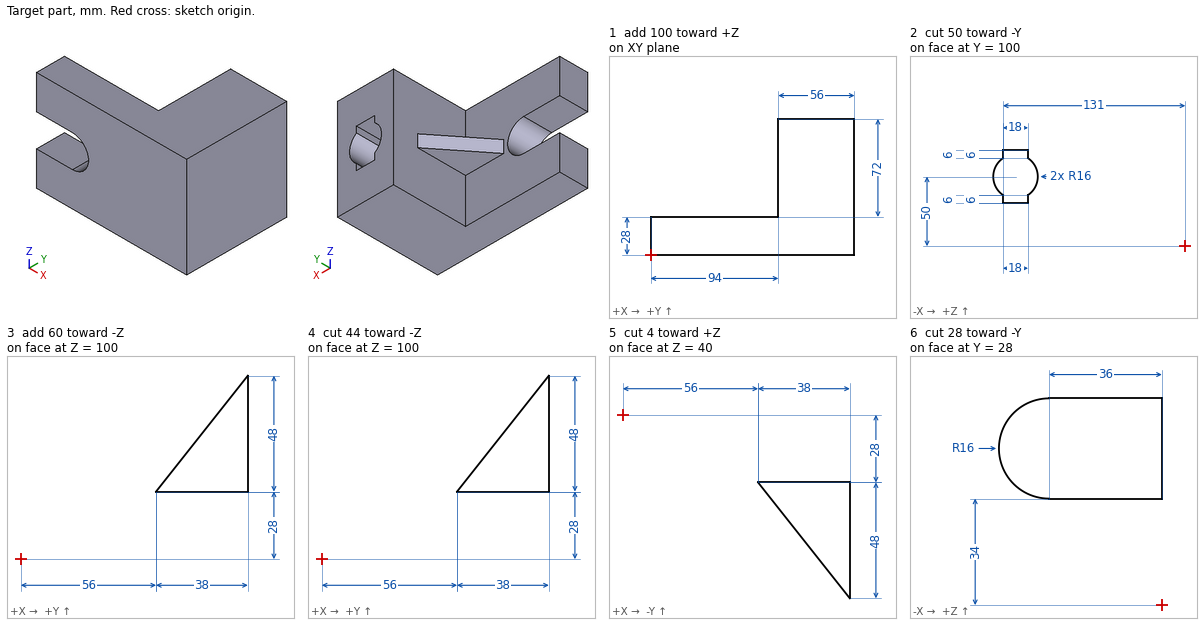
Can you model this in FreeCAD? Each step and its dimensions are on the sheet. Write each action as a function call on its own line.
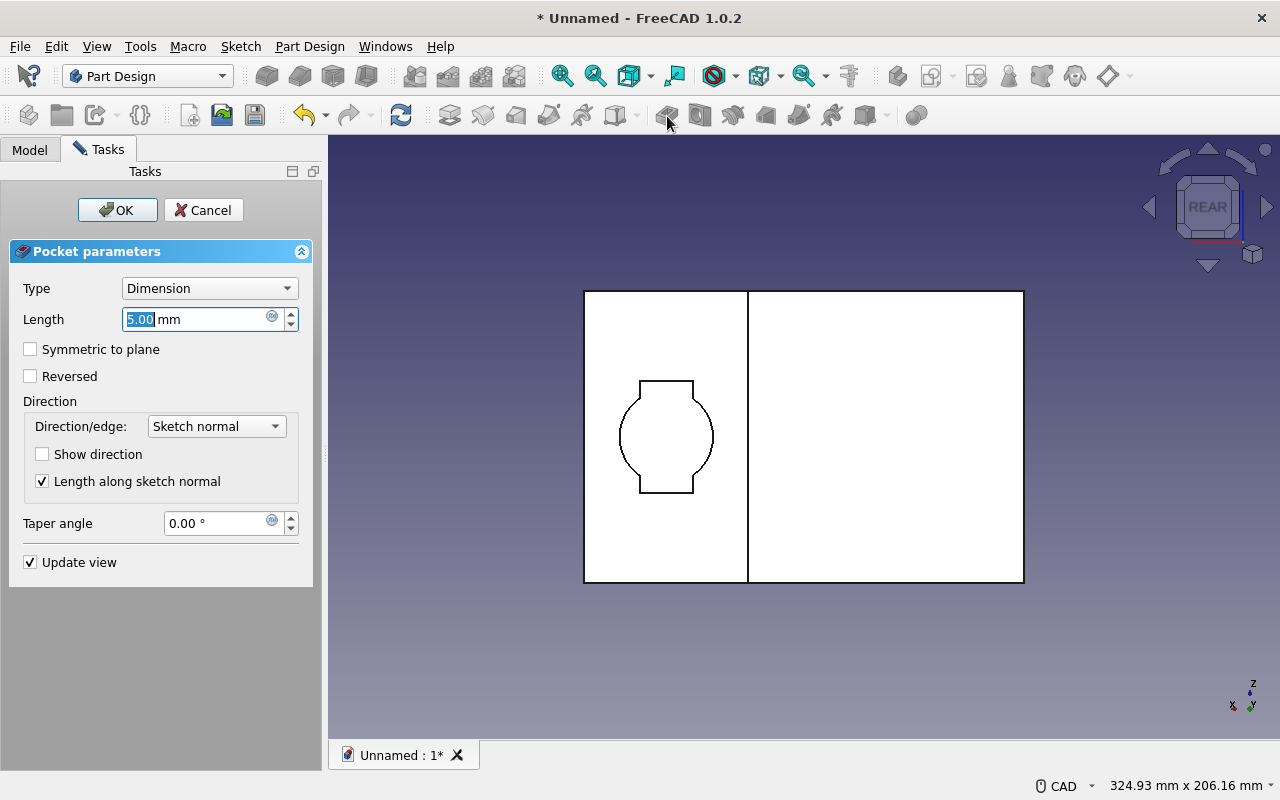
text(50)
key(Tab)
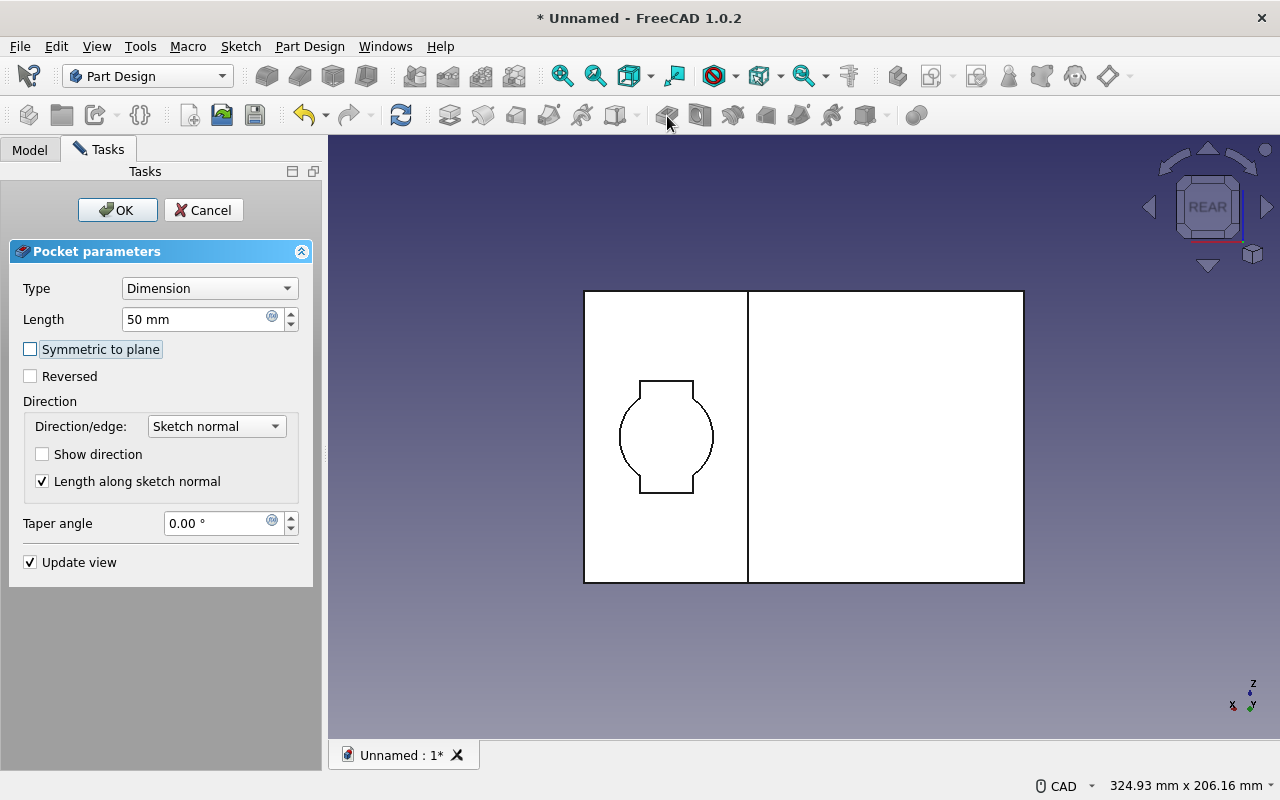
click(118, 210)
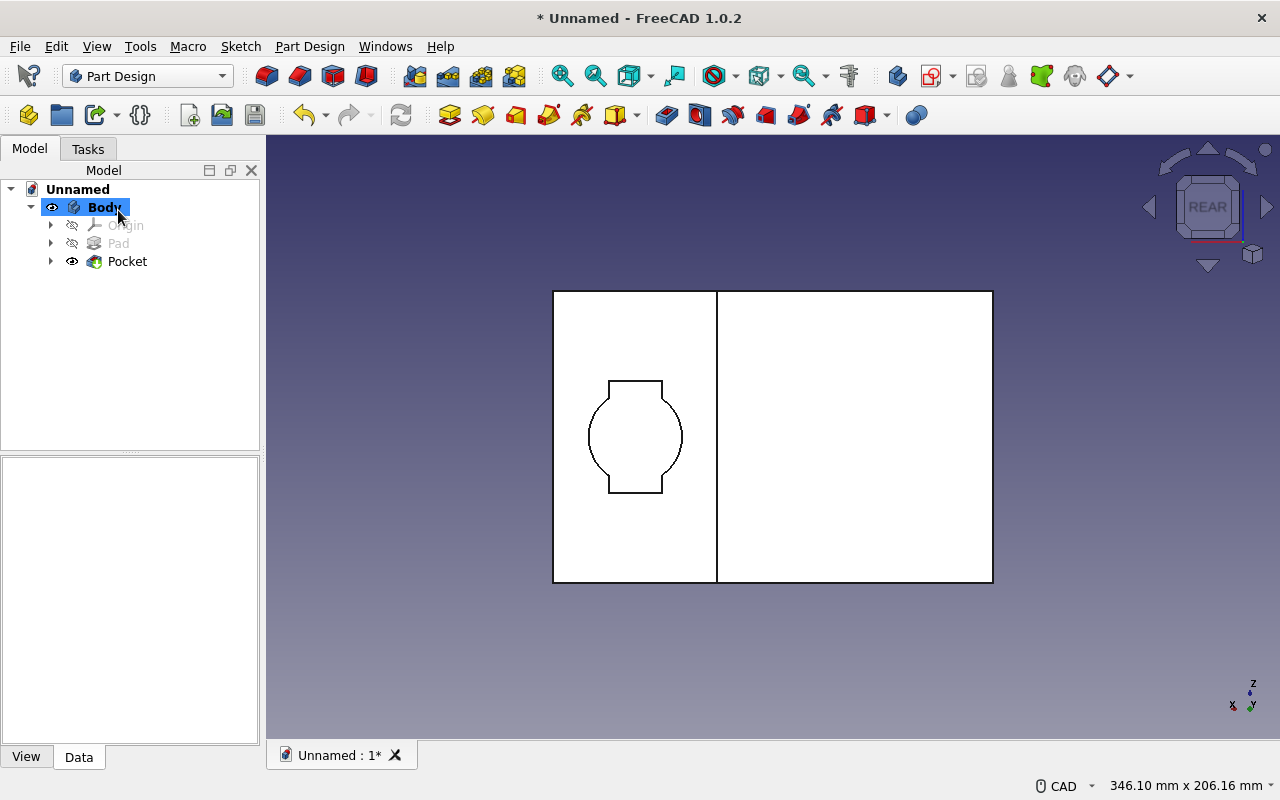
key(0)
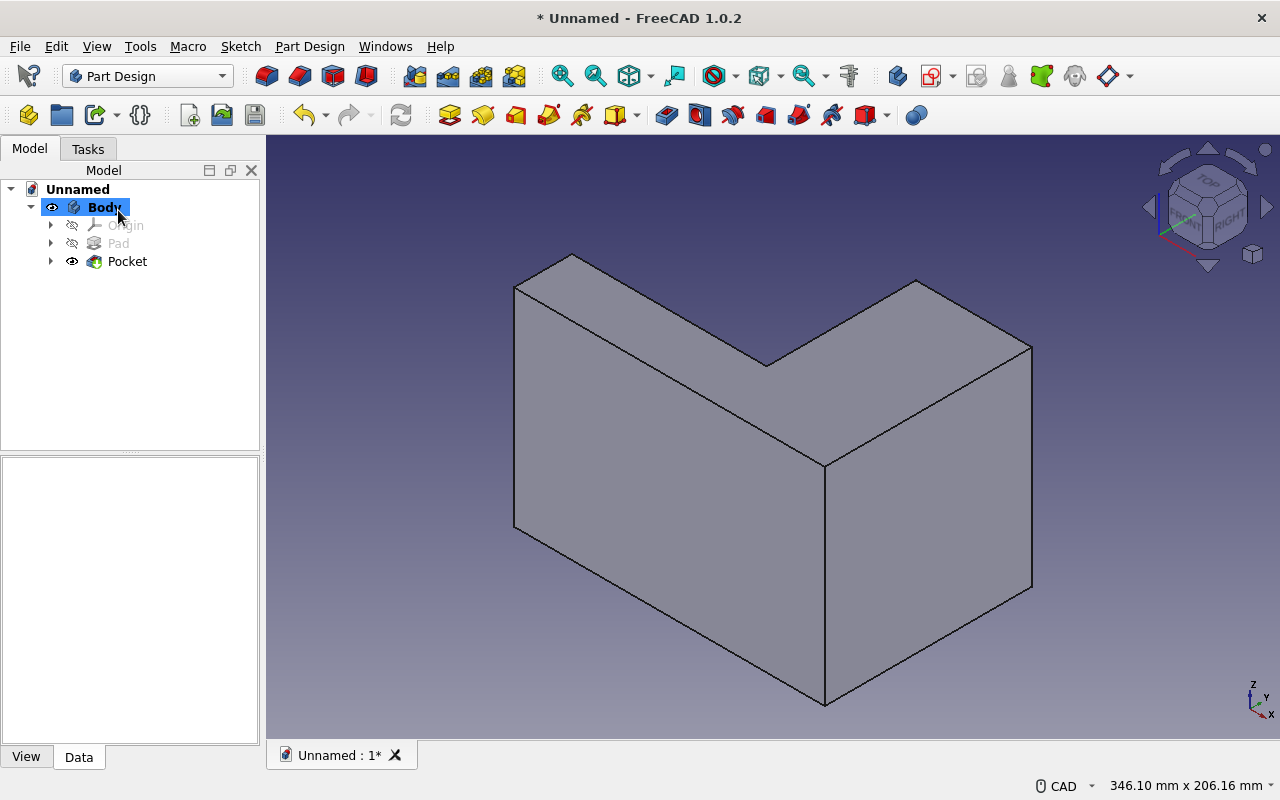
click(891, 351)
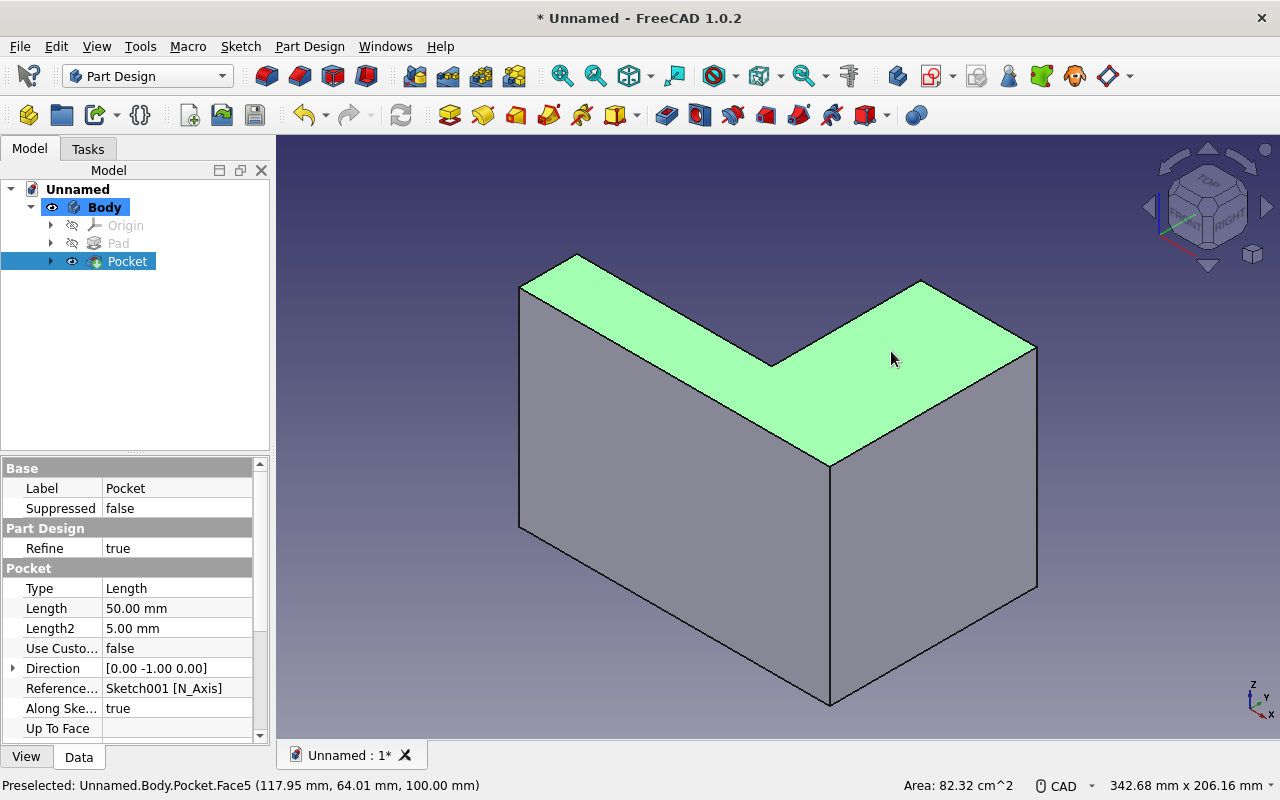
click(930, 76)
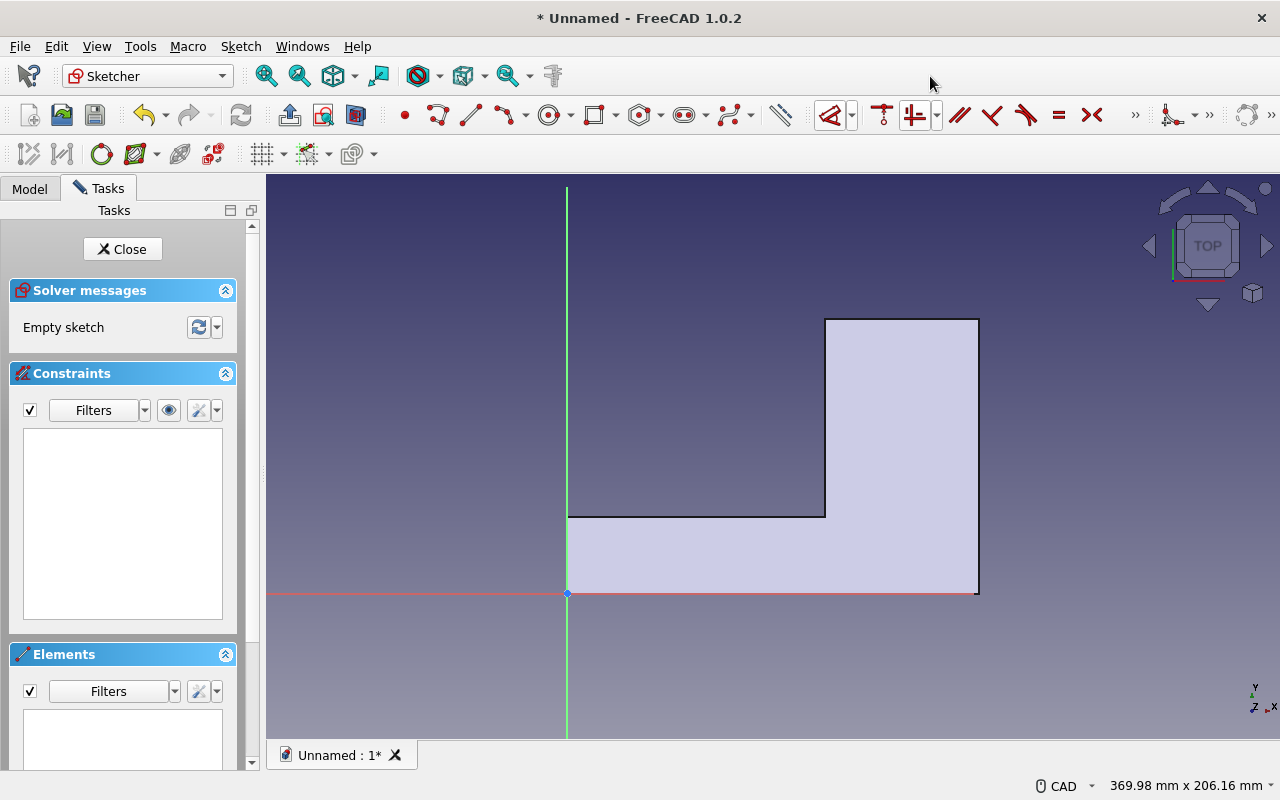
scroll(686, 529, up, 3)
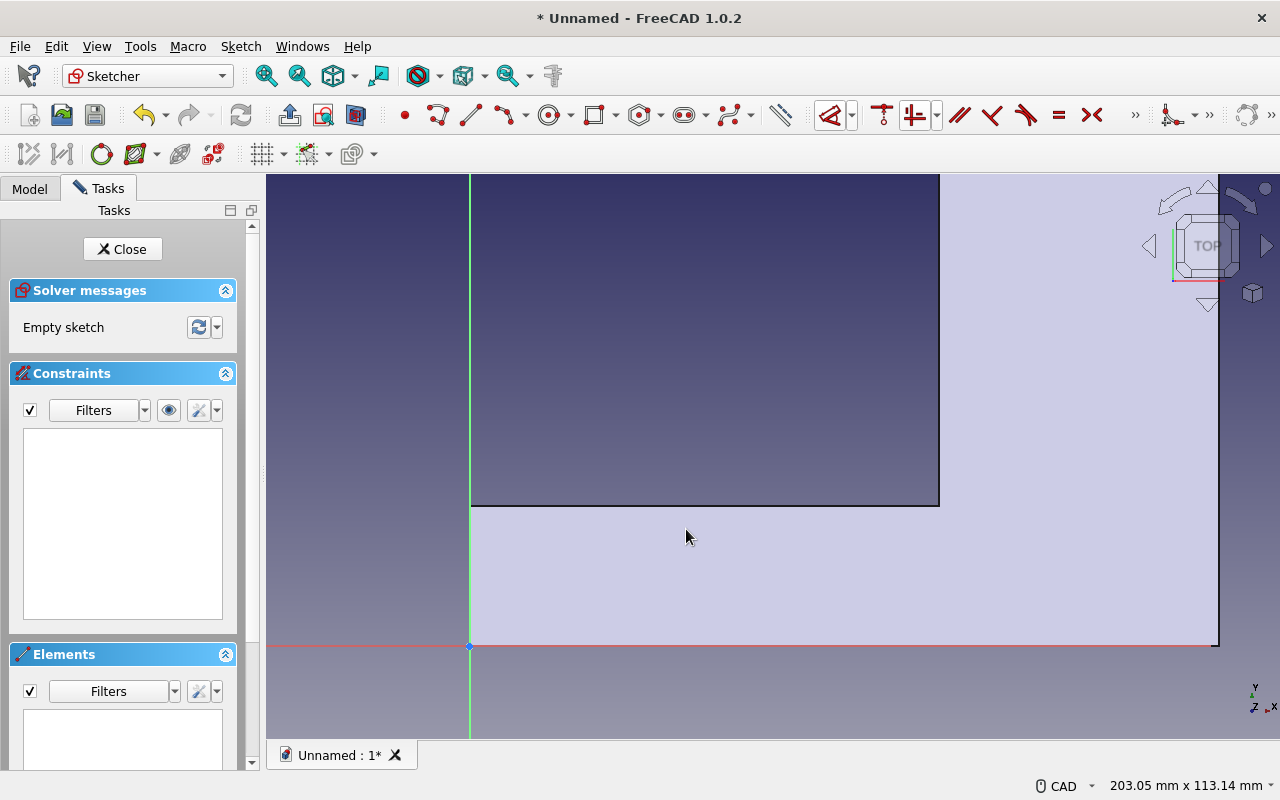
click(438, 116)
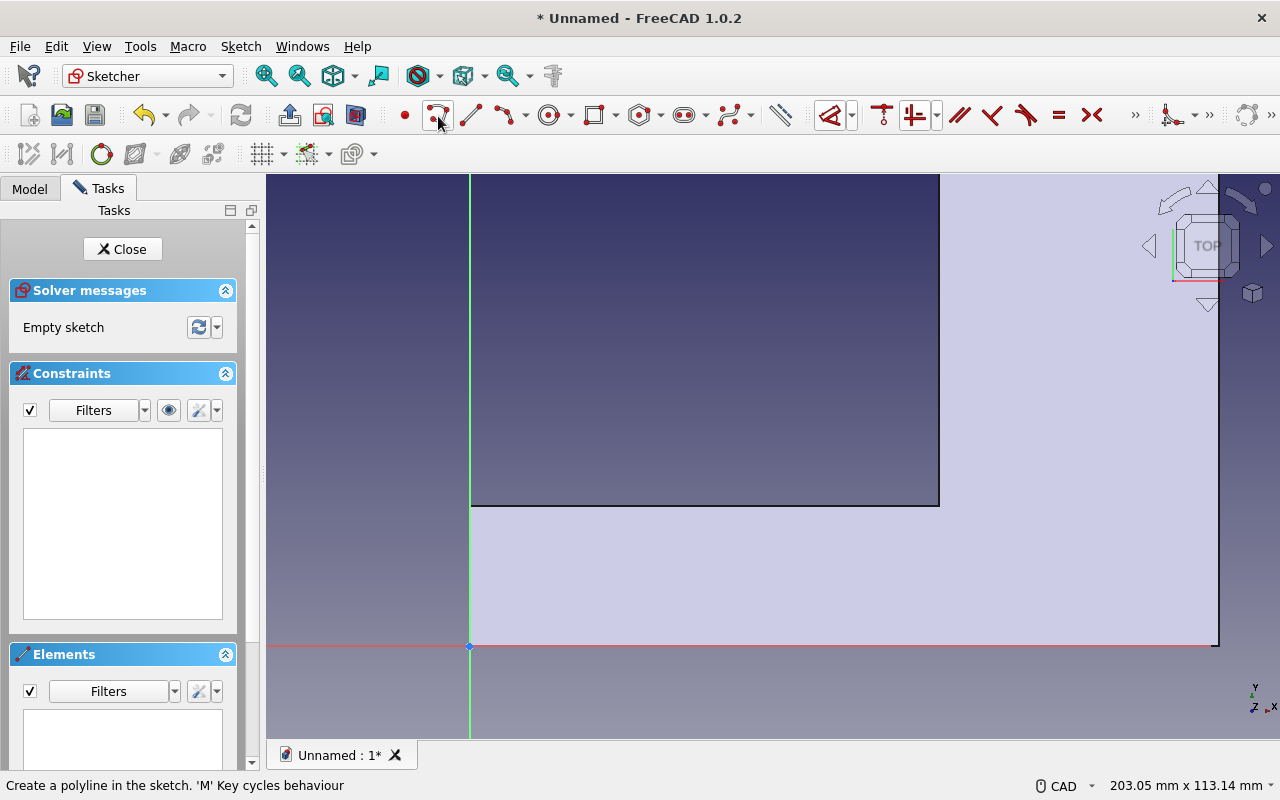
click(749, 506)
click(939, 506)
click(939, 267)
click(749, 507)
key(Escape)
key(Escape)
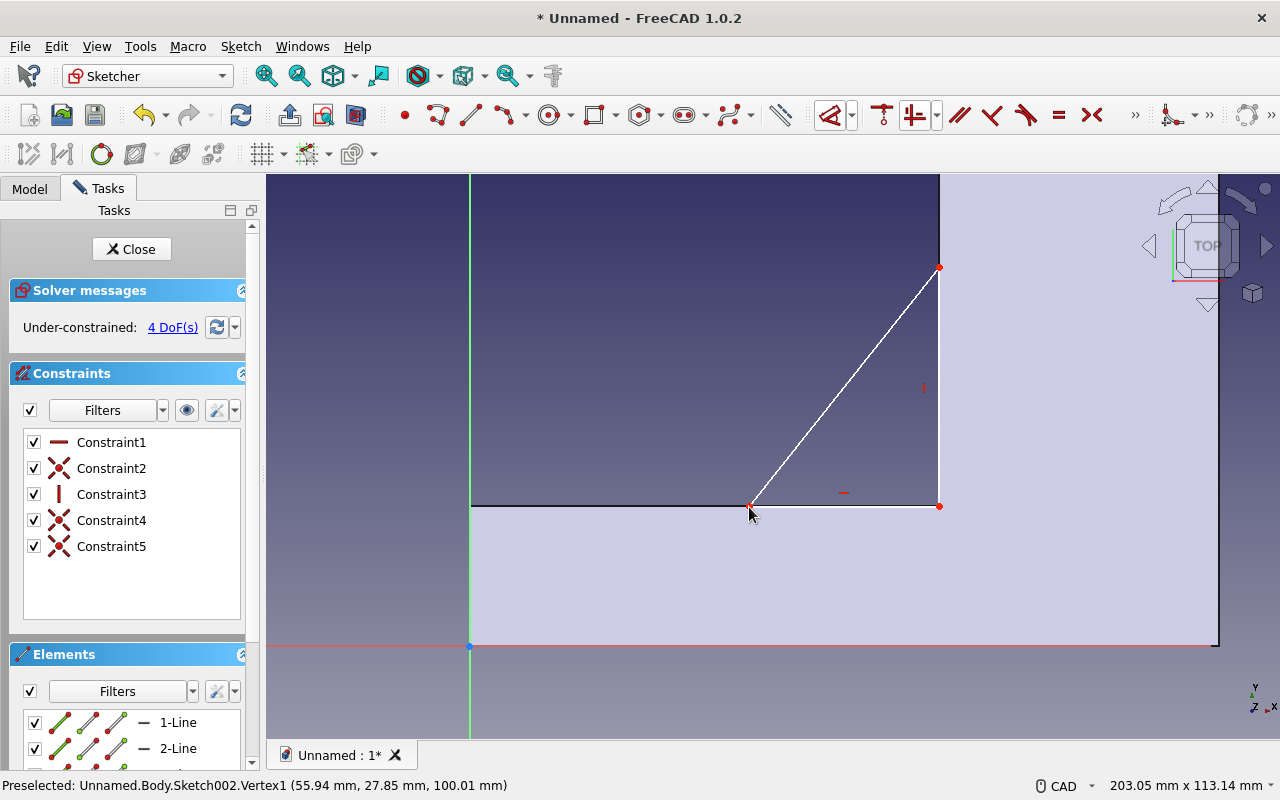
click(806, 507)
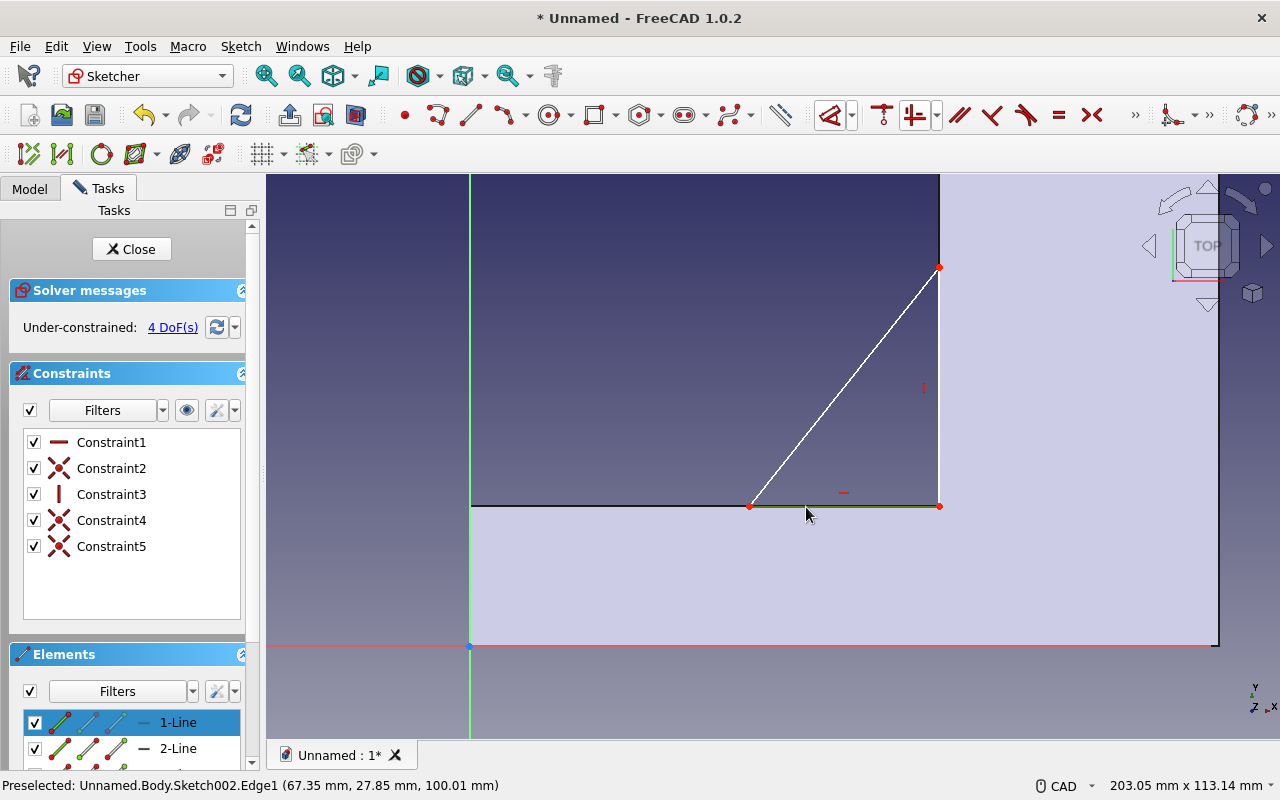
click(852, 116)